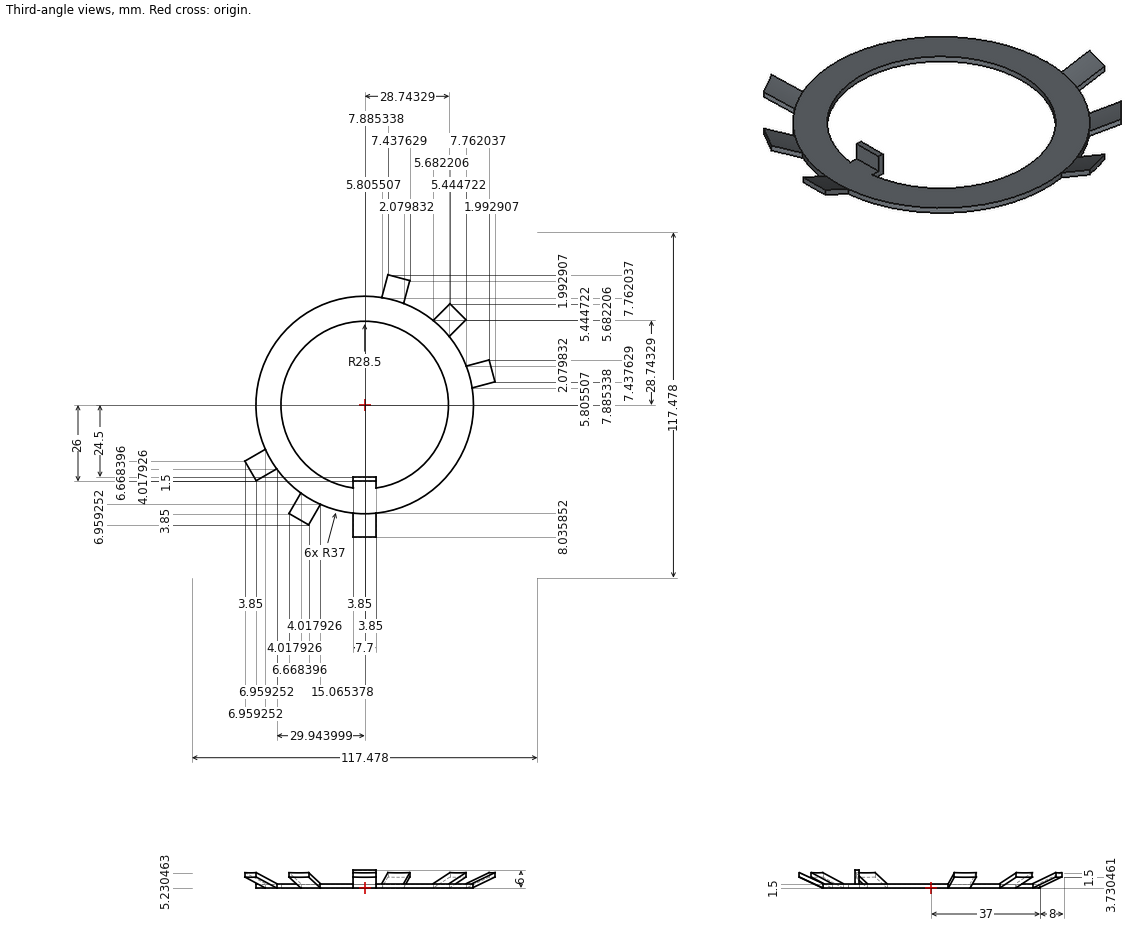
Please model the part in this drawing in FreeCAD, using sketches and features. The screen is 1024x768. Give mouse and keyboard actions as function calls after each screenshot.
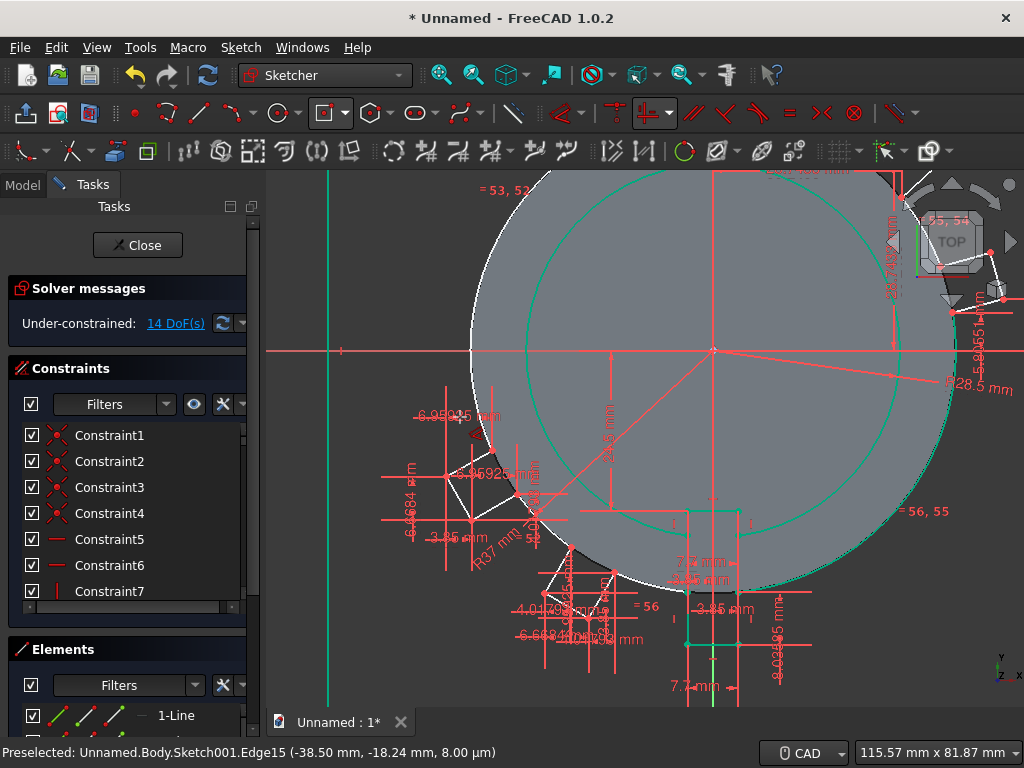
scroll(465, 510, down, 4)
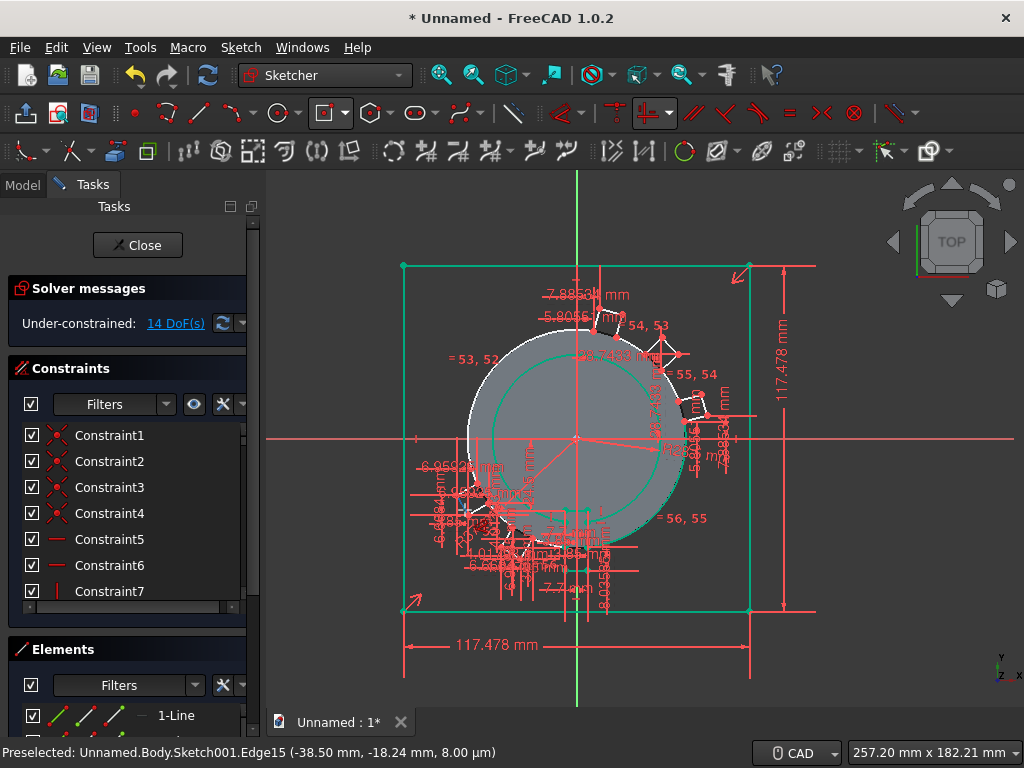
scroll(596, 324, up, 4)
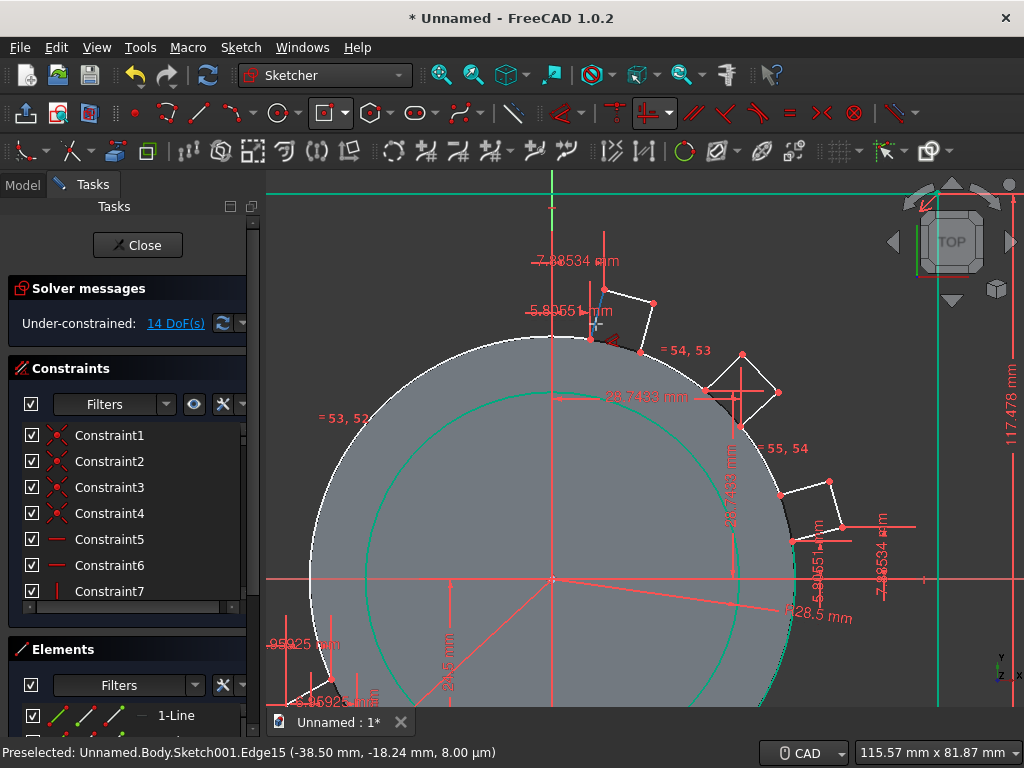
click(595, 325)
click(662, 326)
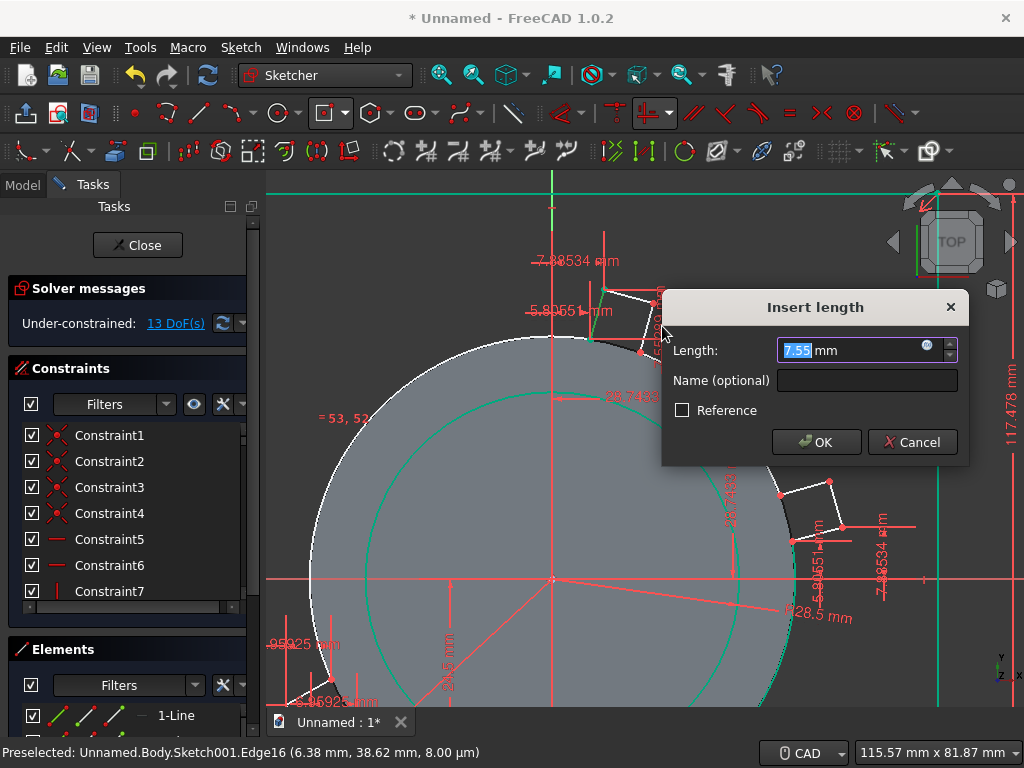
text(7.762037)
key(Return)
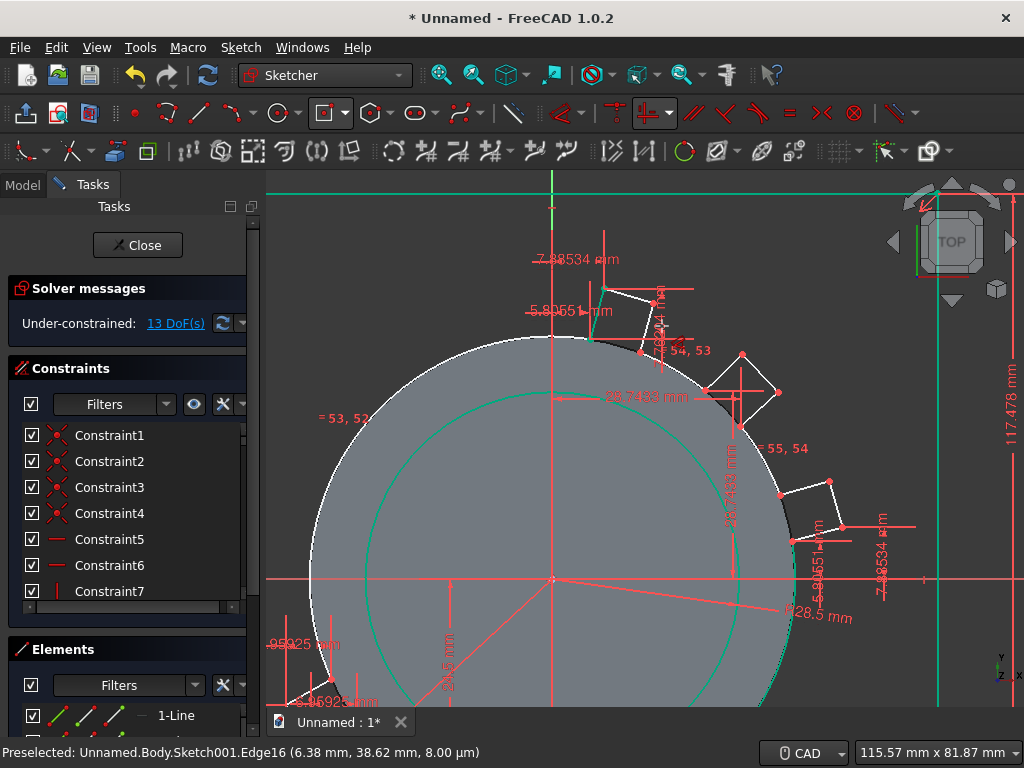
click(619, 293)
click(629, 231)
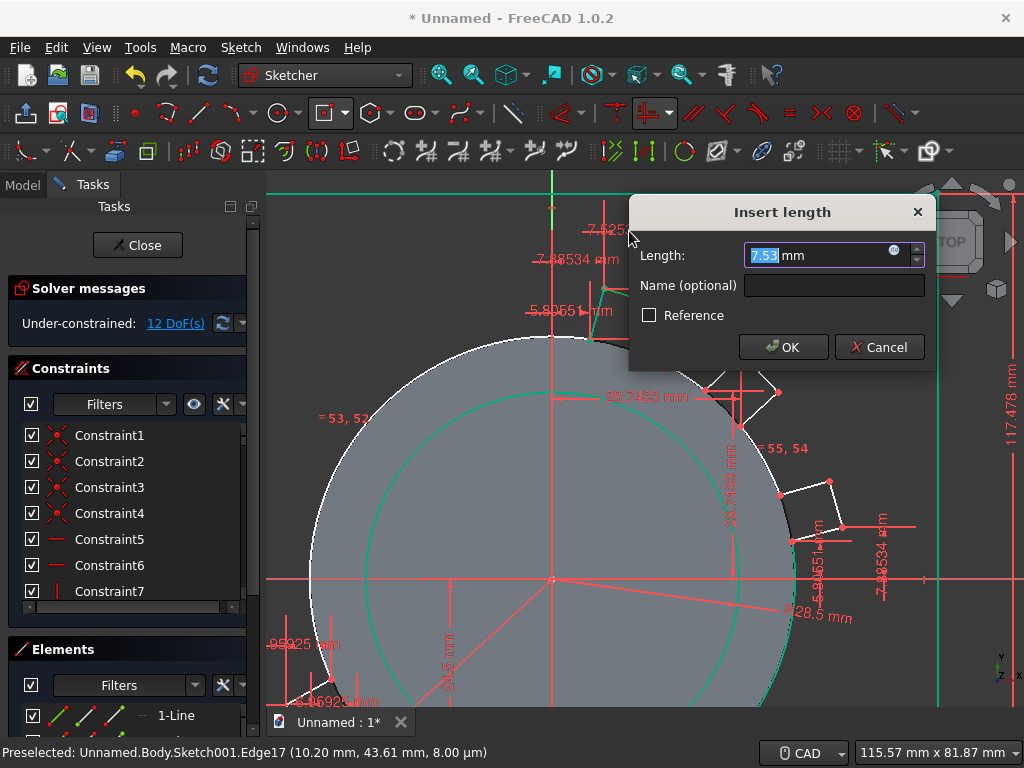
text(7.437629)
key(Return)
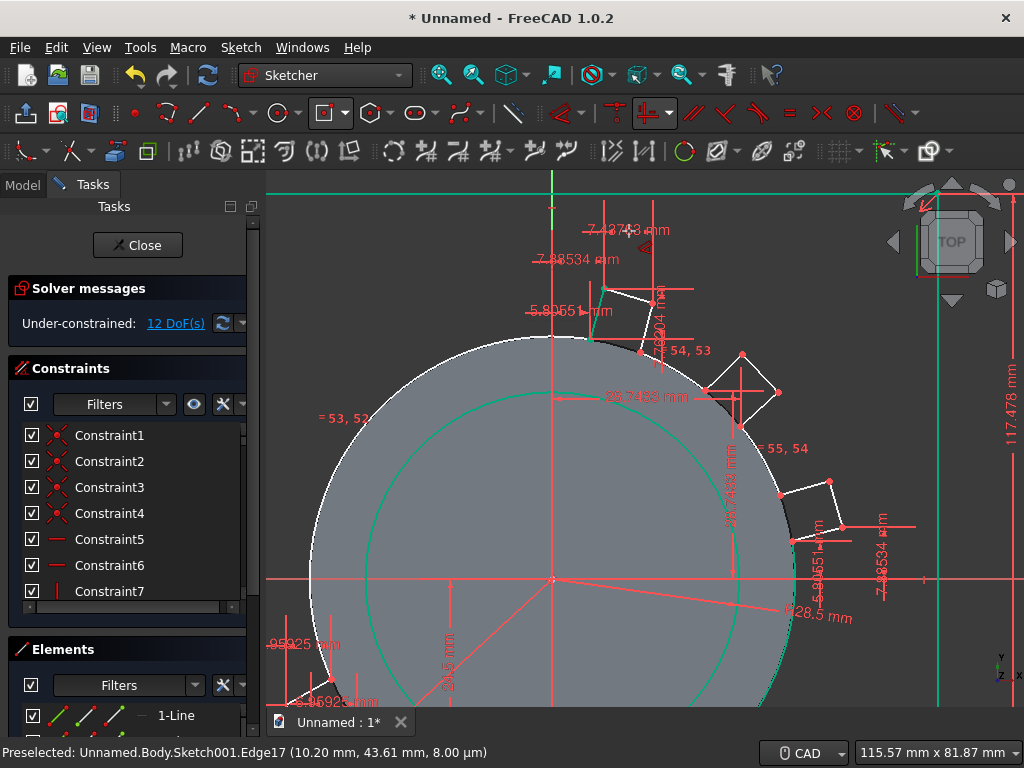
scroll(619, 293, up, 6)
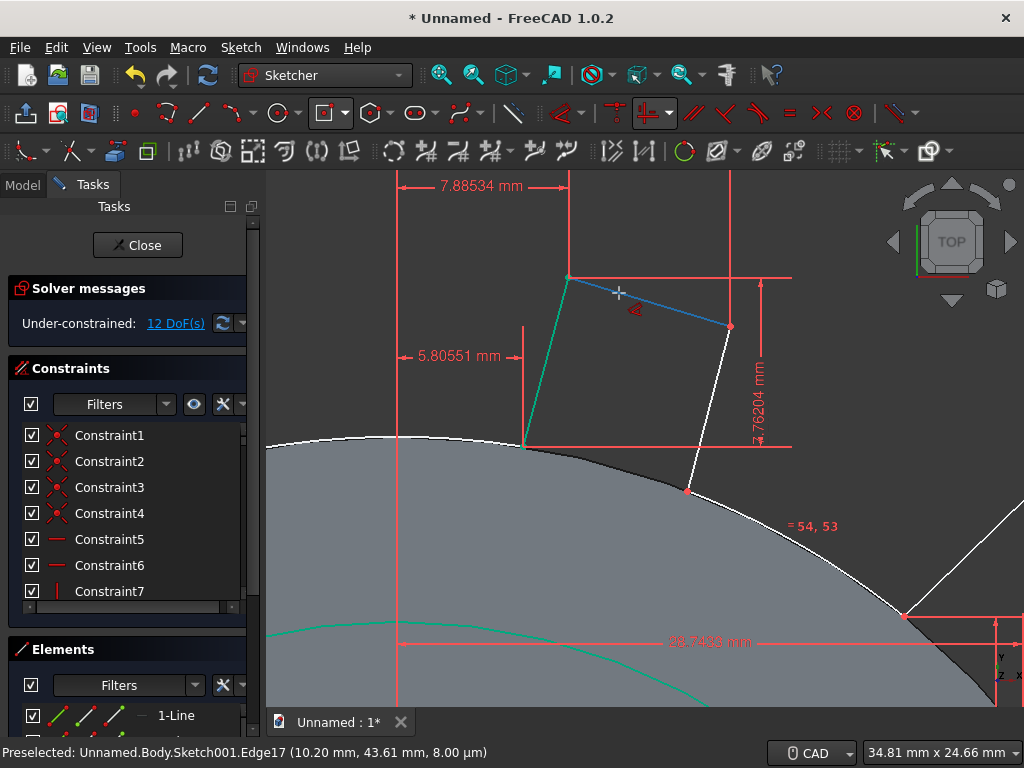
click(617, 292)
click(764, 302)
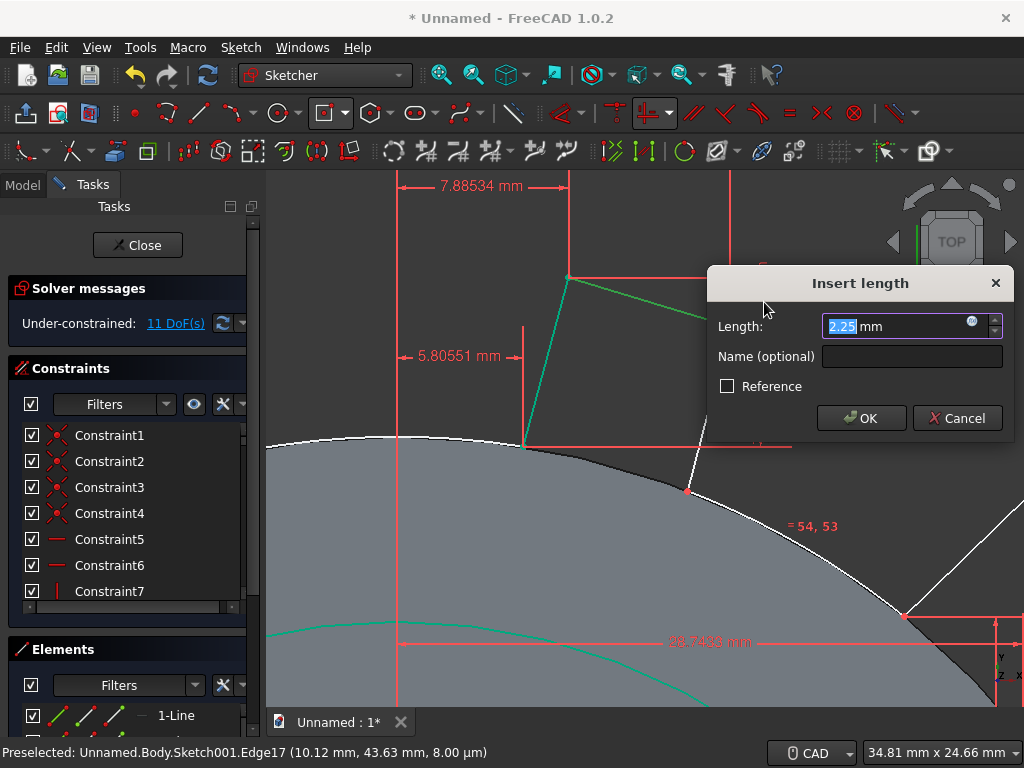
text(1.992907)
key(Return)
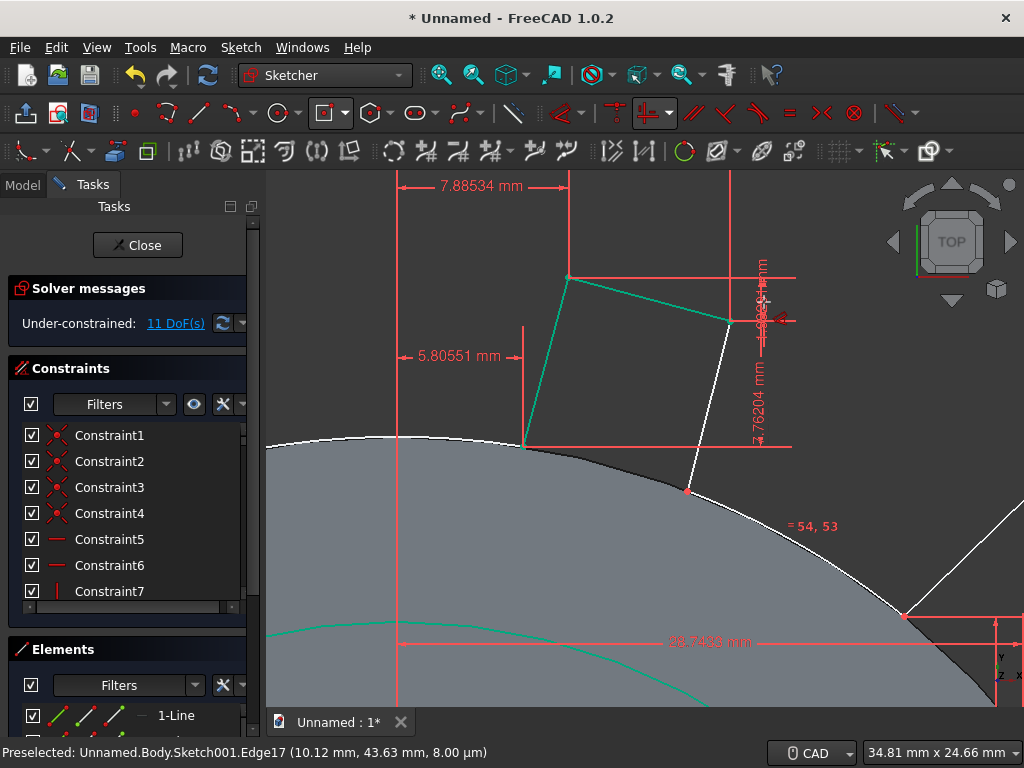
click(718, 372)
click(694, 287)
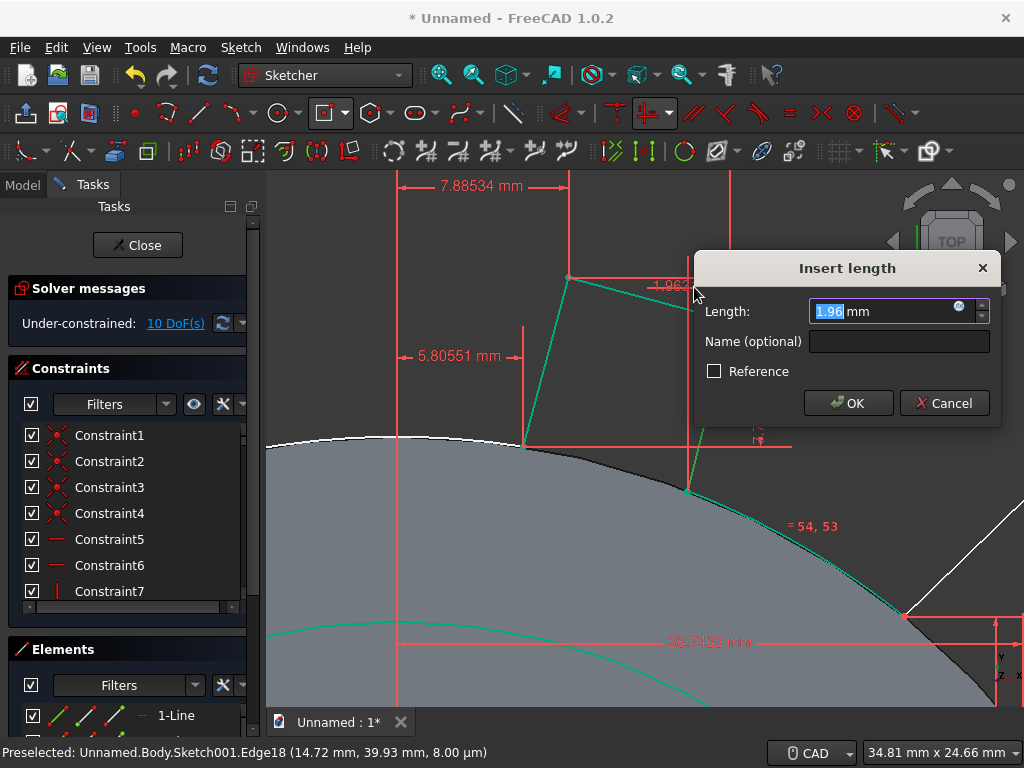
text(2.079832)
key(Return)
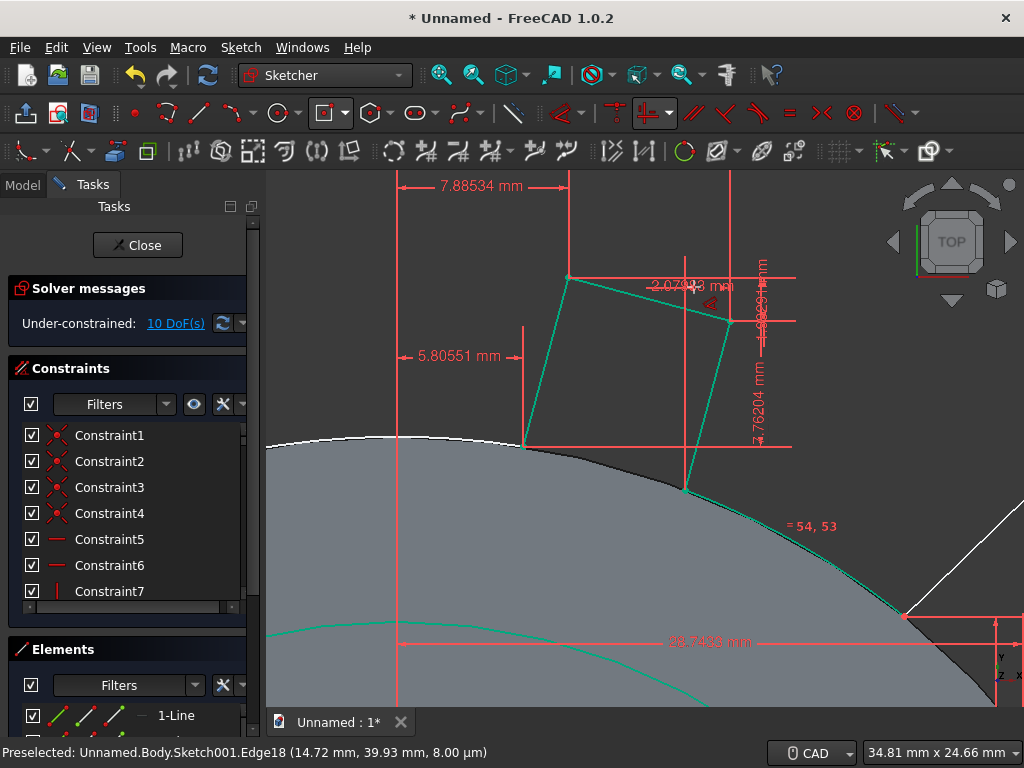
scroll(605, 313, down, 10)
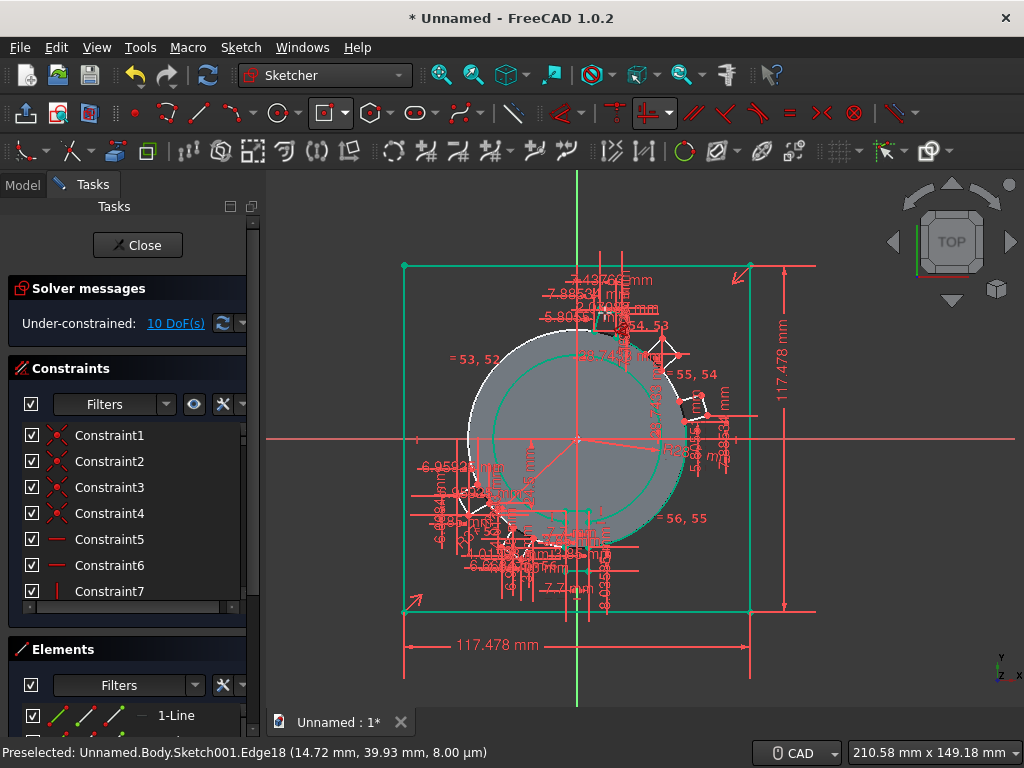
scroll(651, 349, up, 5)